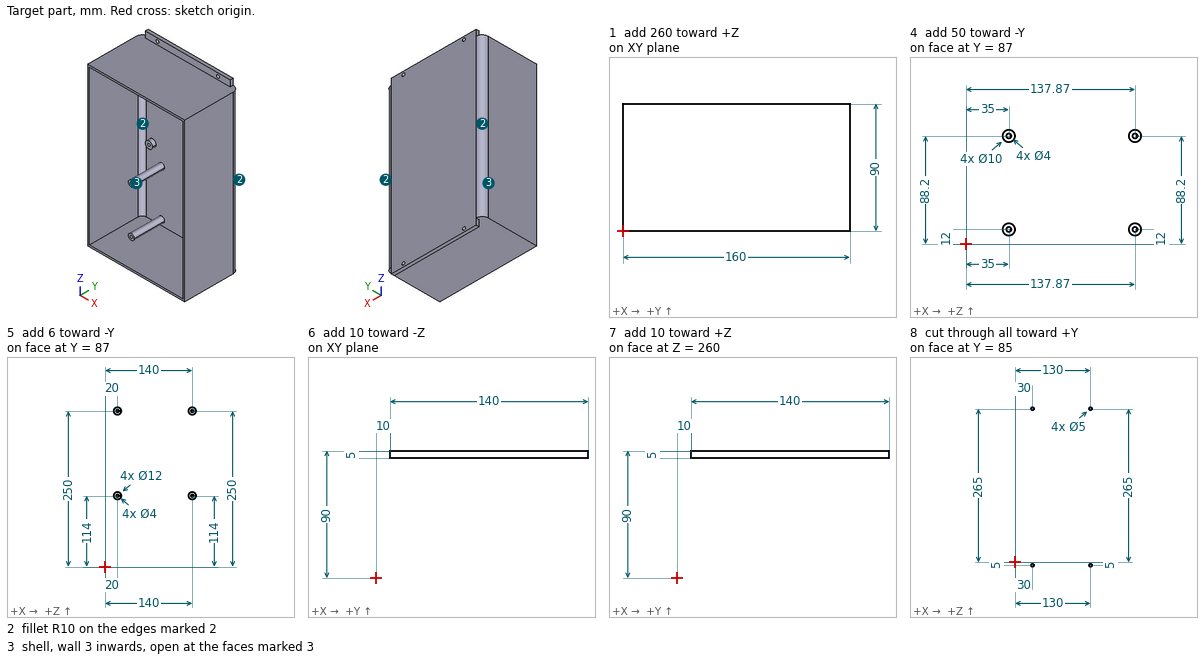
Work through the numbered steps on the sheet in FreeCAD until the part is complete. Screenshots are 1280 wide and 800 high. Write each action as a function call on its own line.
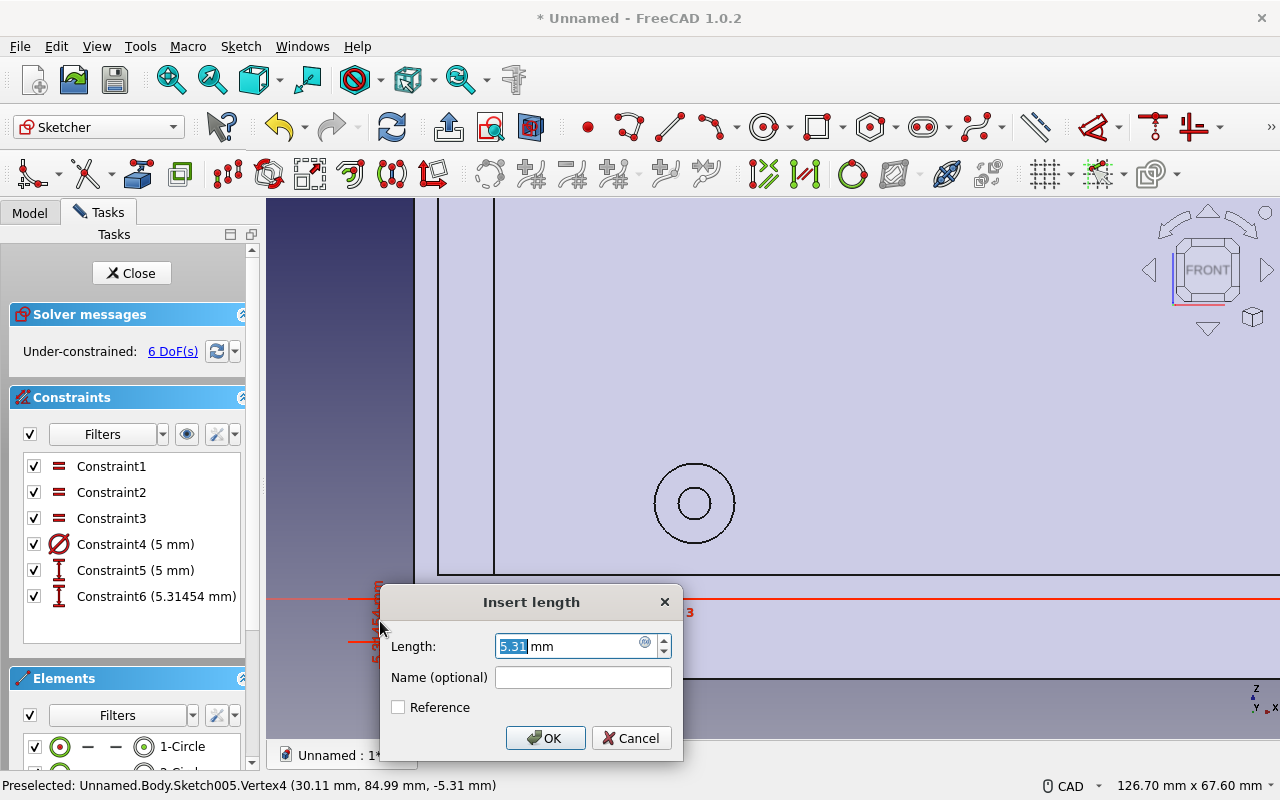
text(5)
key(Return)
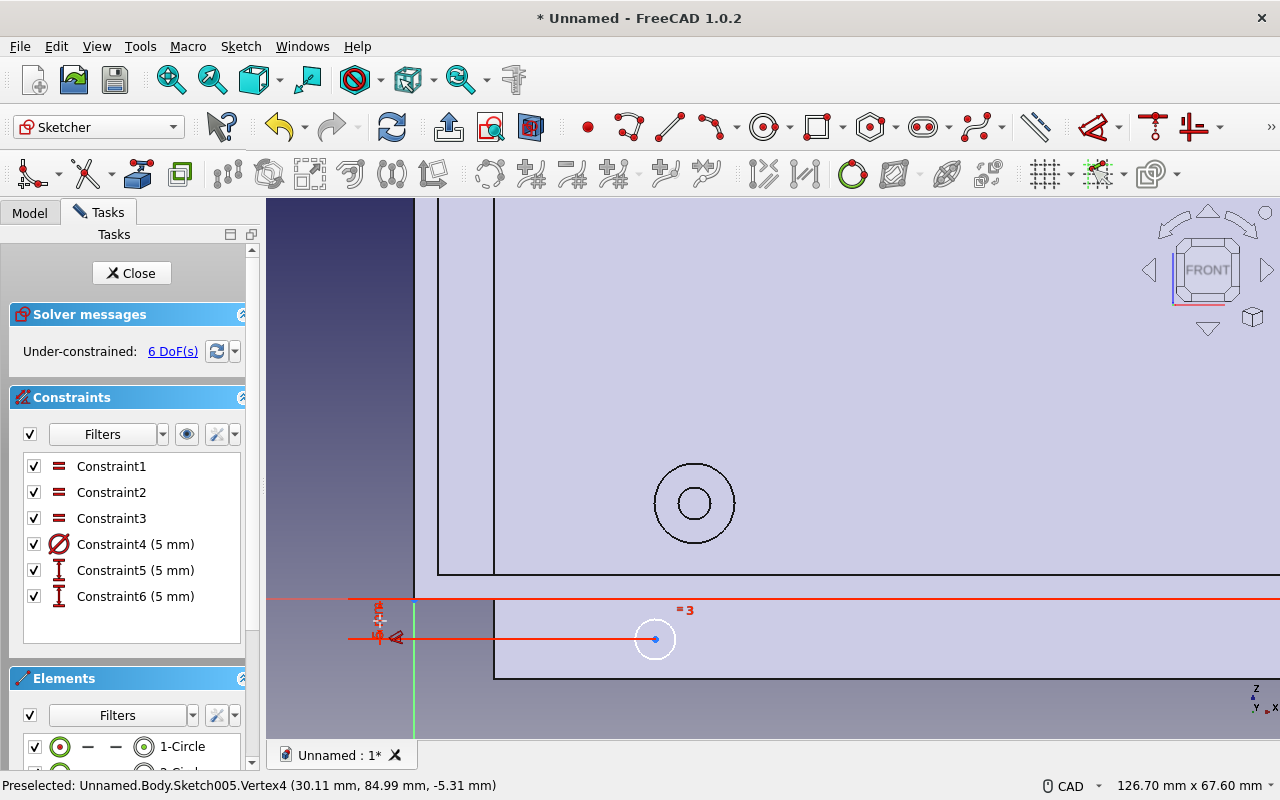
scroll(657, 649, down, 9)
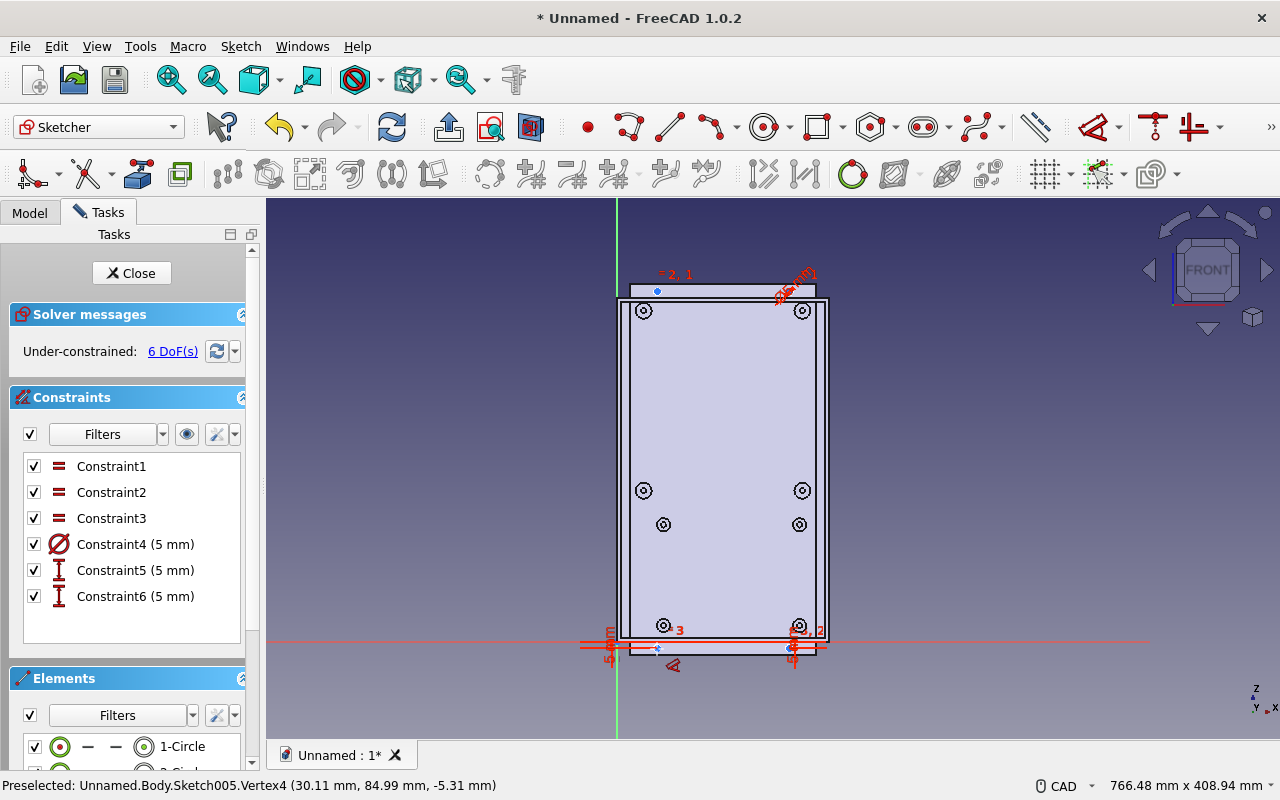
click(657, 292)
click(637, 258)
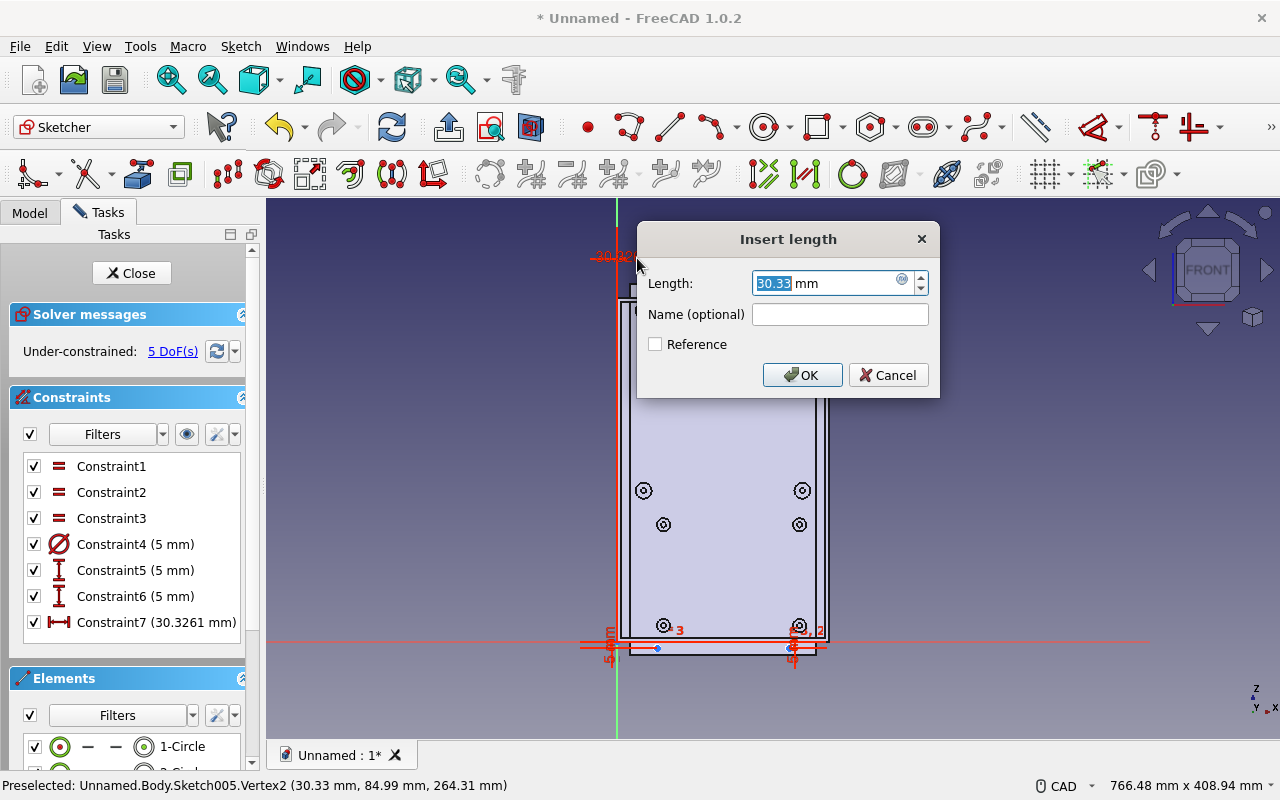
text(30)
key(Return)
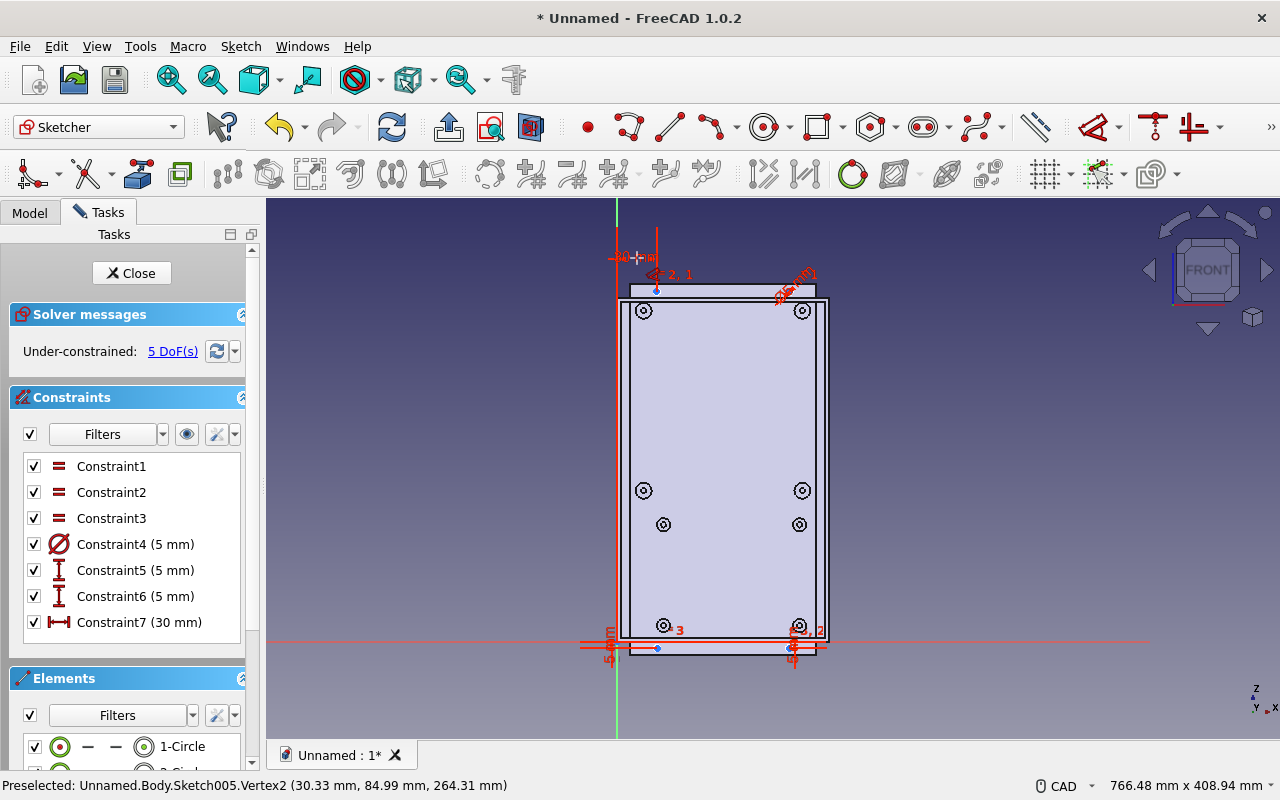
click(657, 648)
click(637, 682)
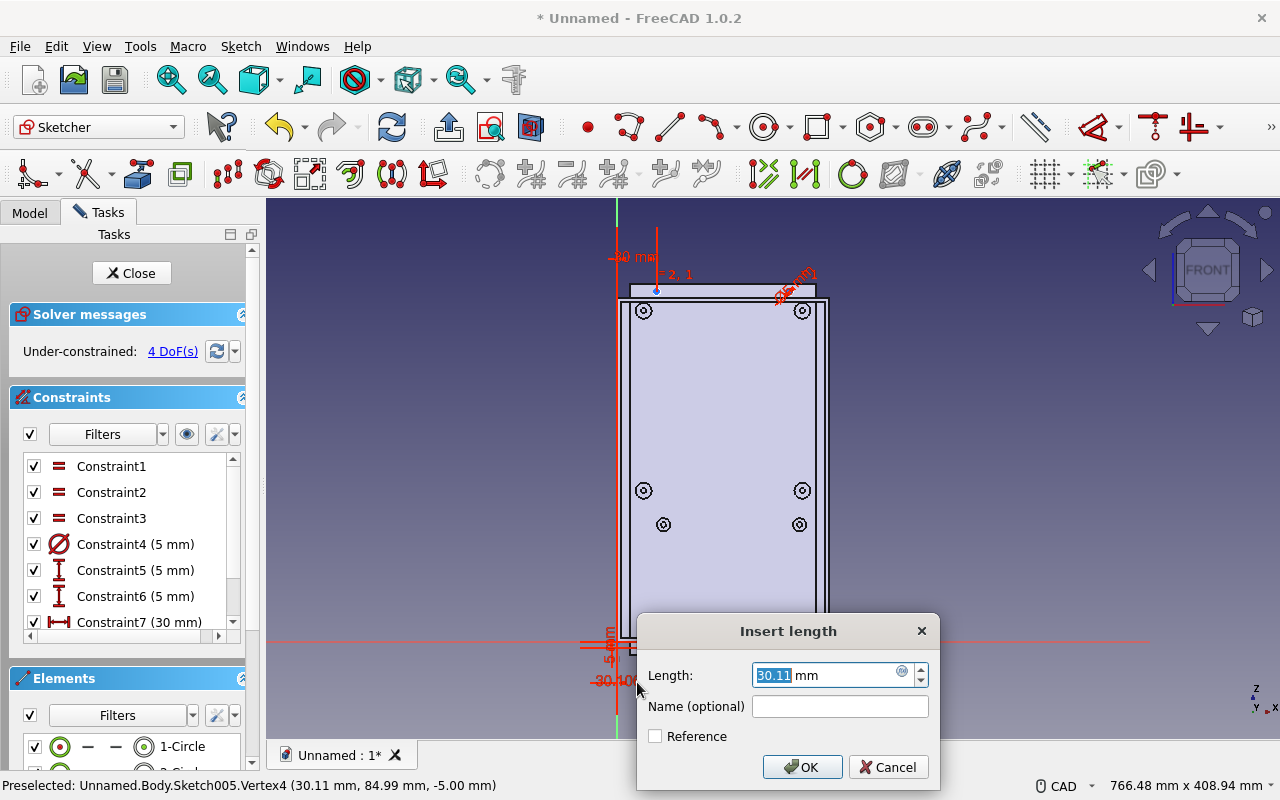
text(30)
key(Return)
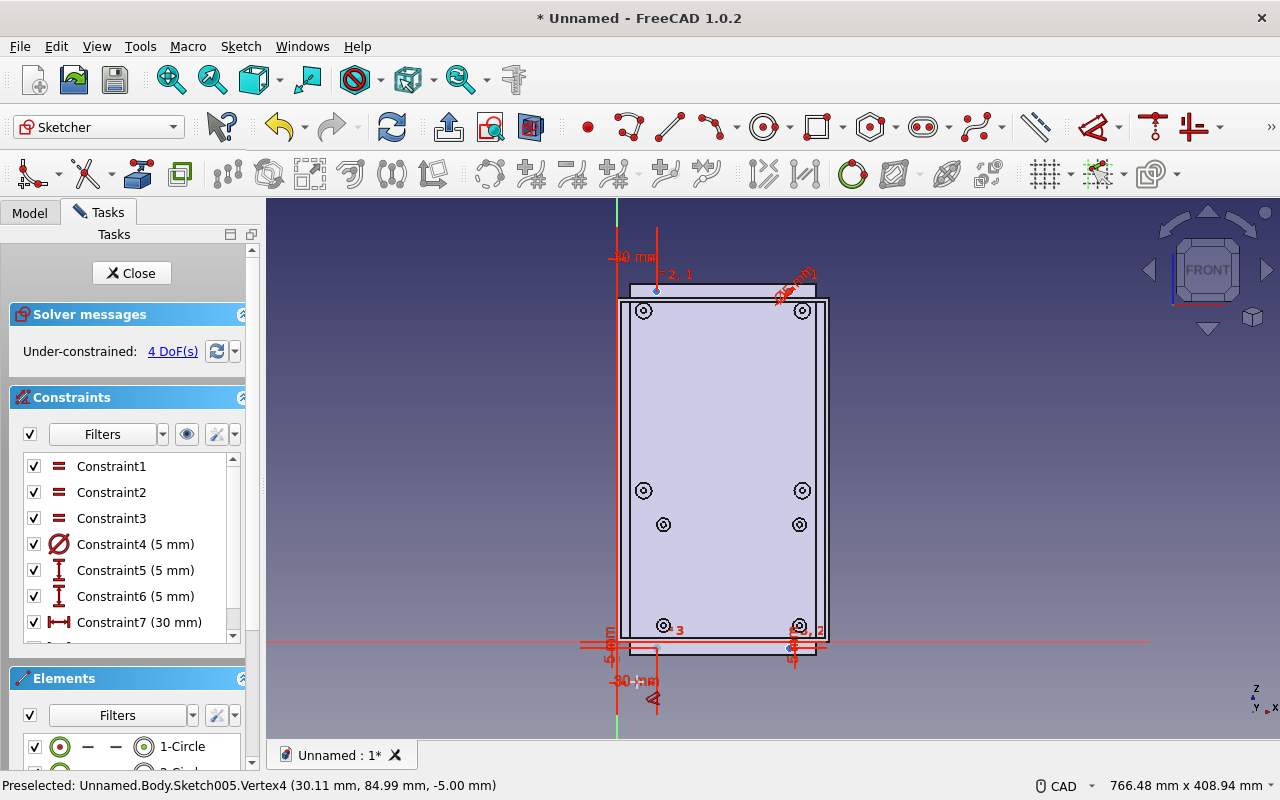
click(790, 292)
click(743, 258)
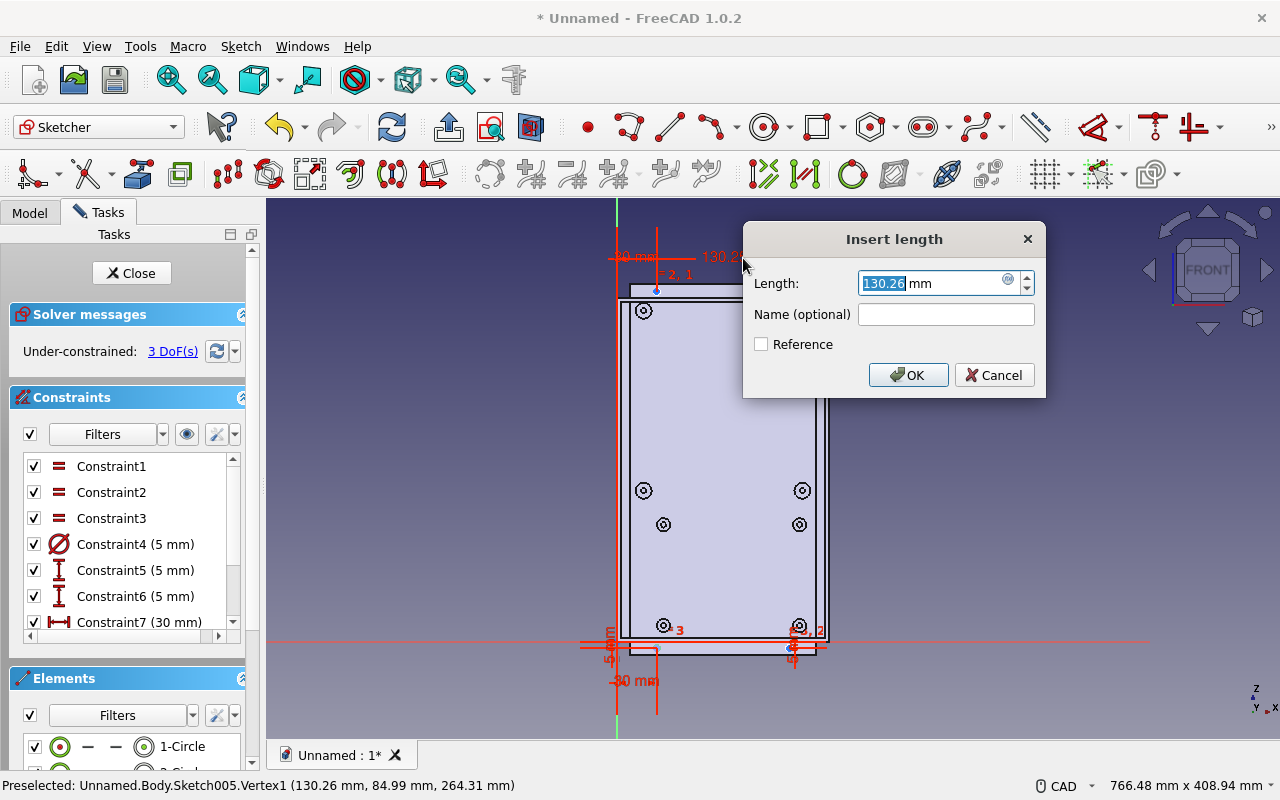
text(130)
key(Return)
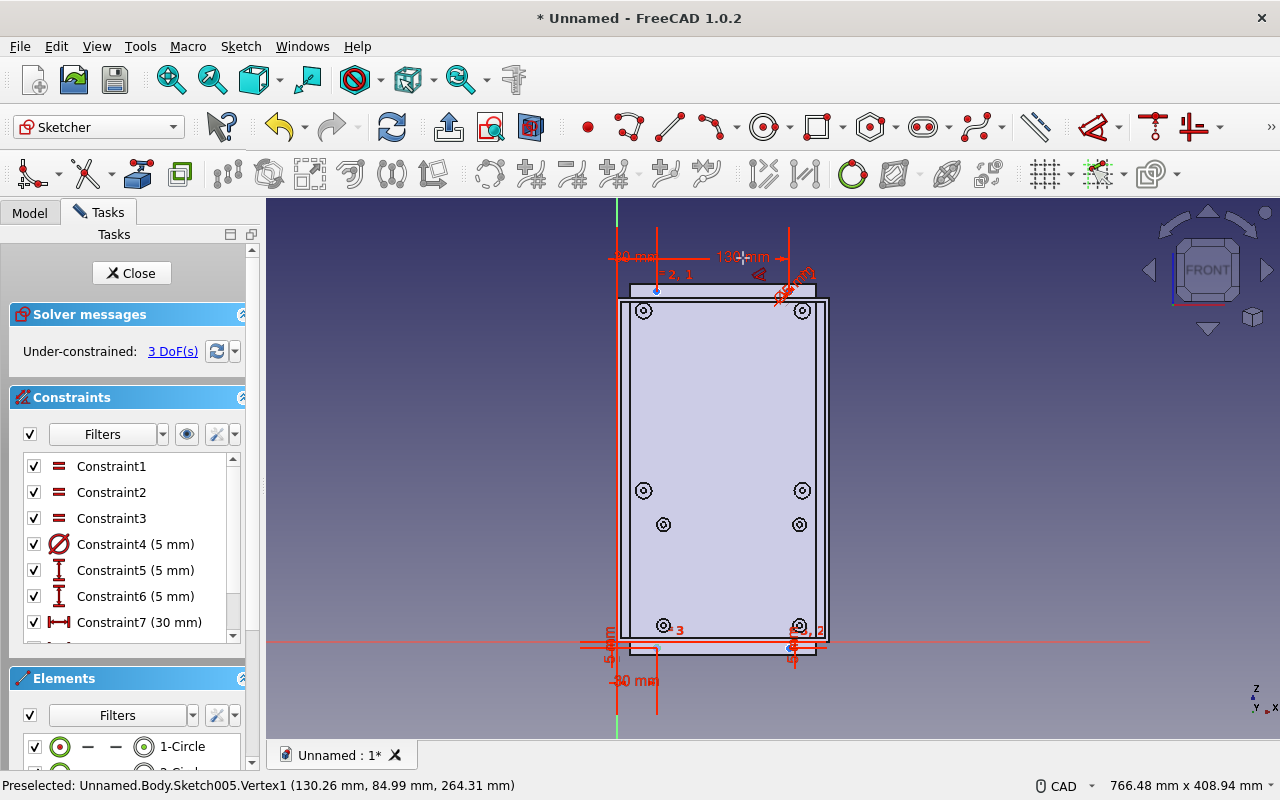
click(789, 292)
click(583, 467)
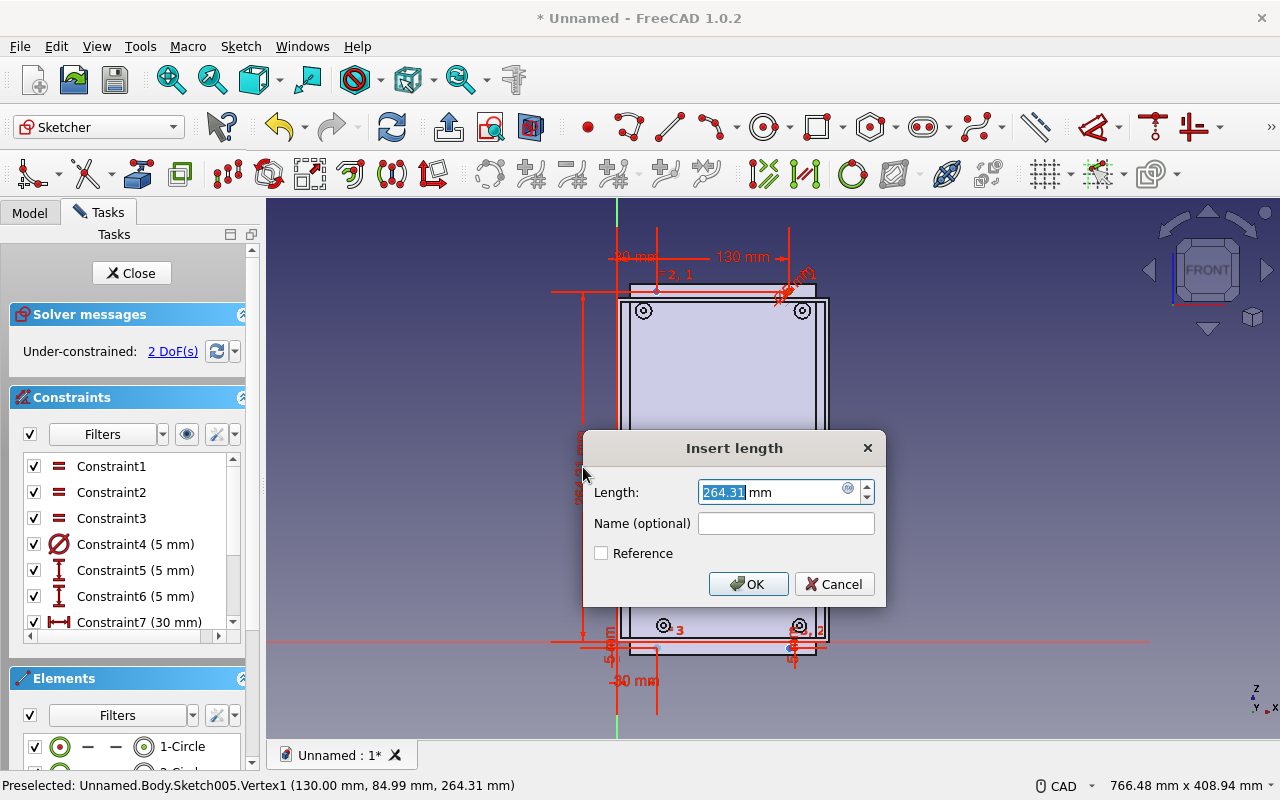
text(265)
key(Return)